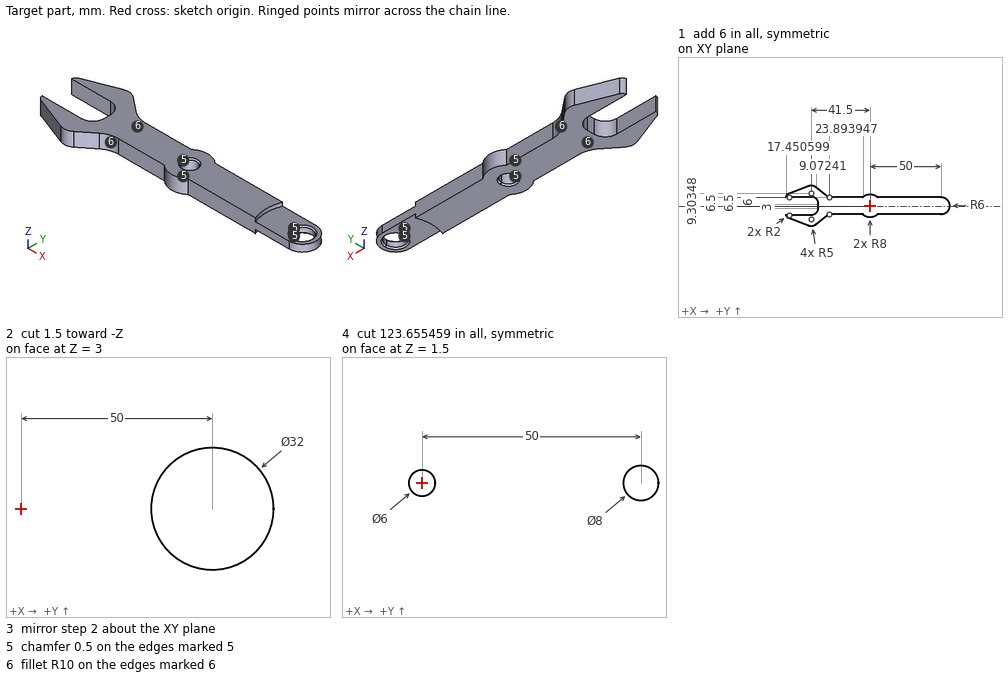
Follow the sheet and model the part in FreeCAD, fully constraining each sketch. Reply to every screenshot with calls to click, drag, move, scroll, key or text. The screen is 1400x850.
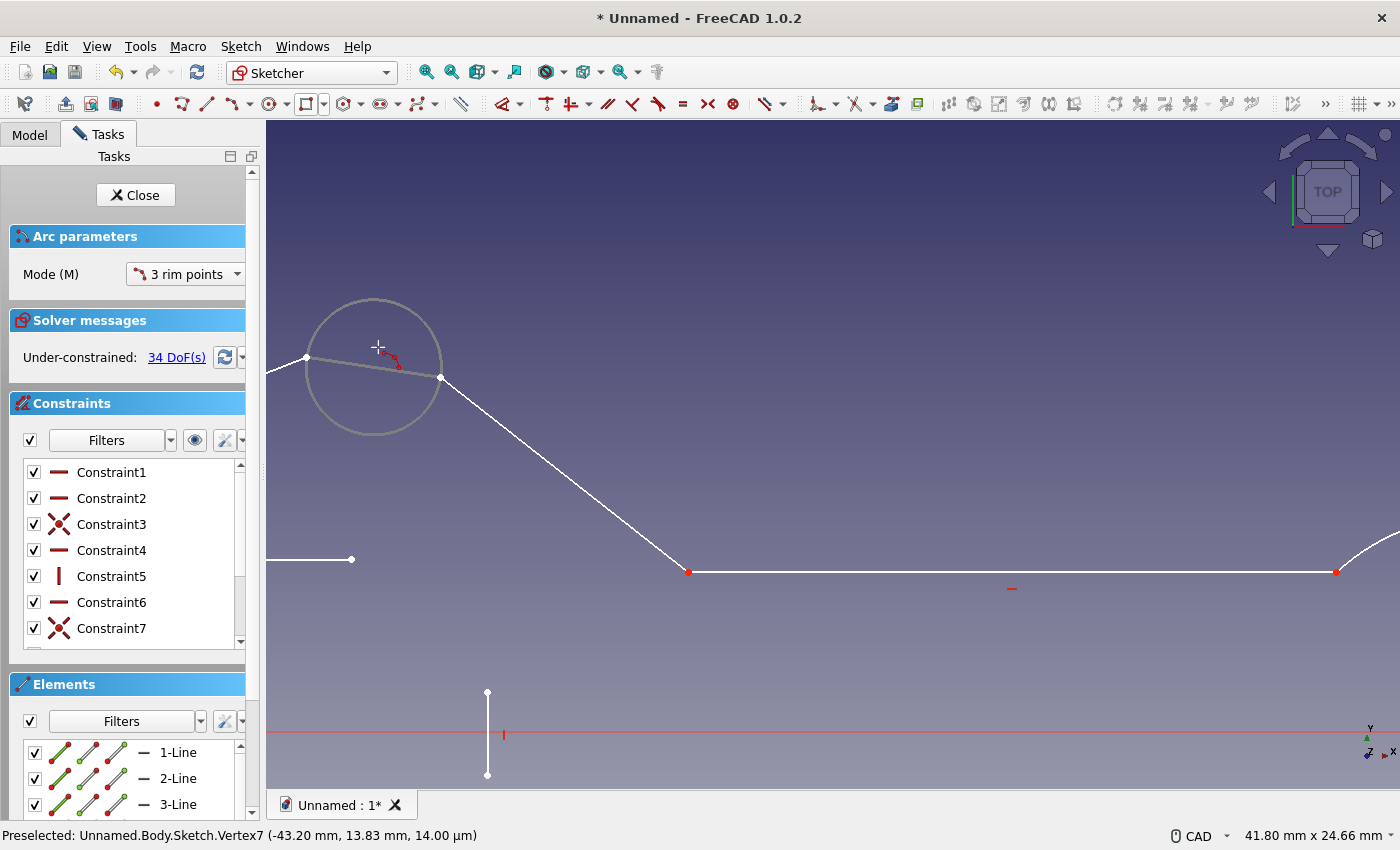
click(377, 346)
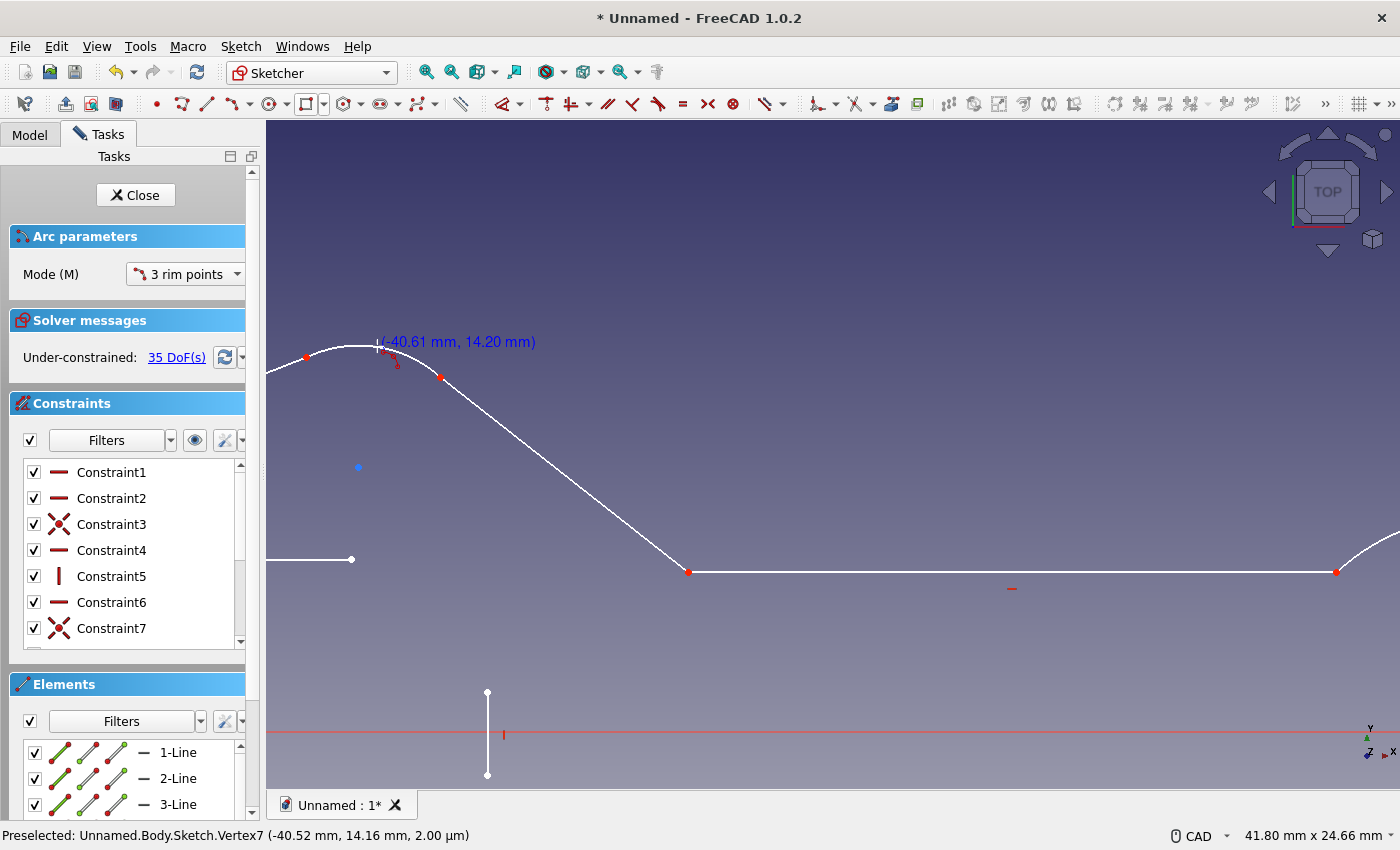
scroll(594, 384, down, 8)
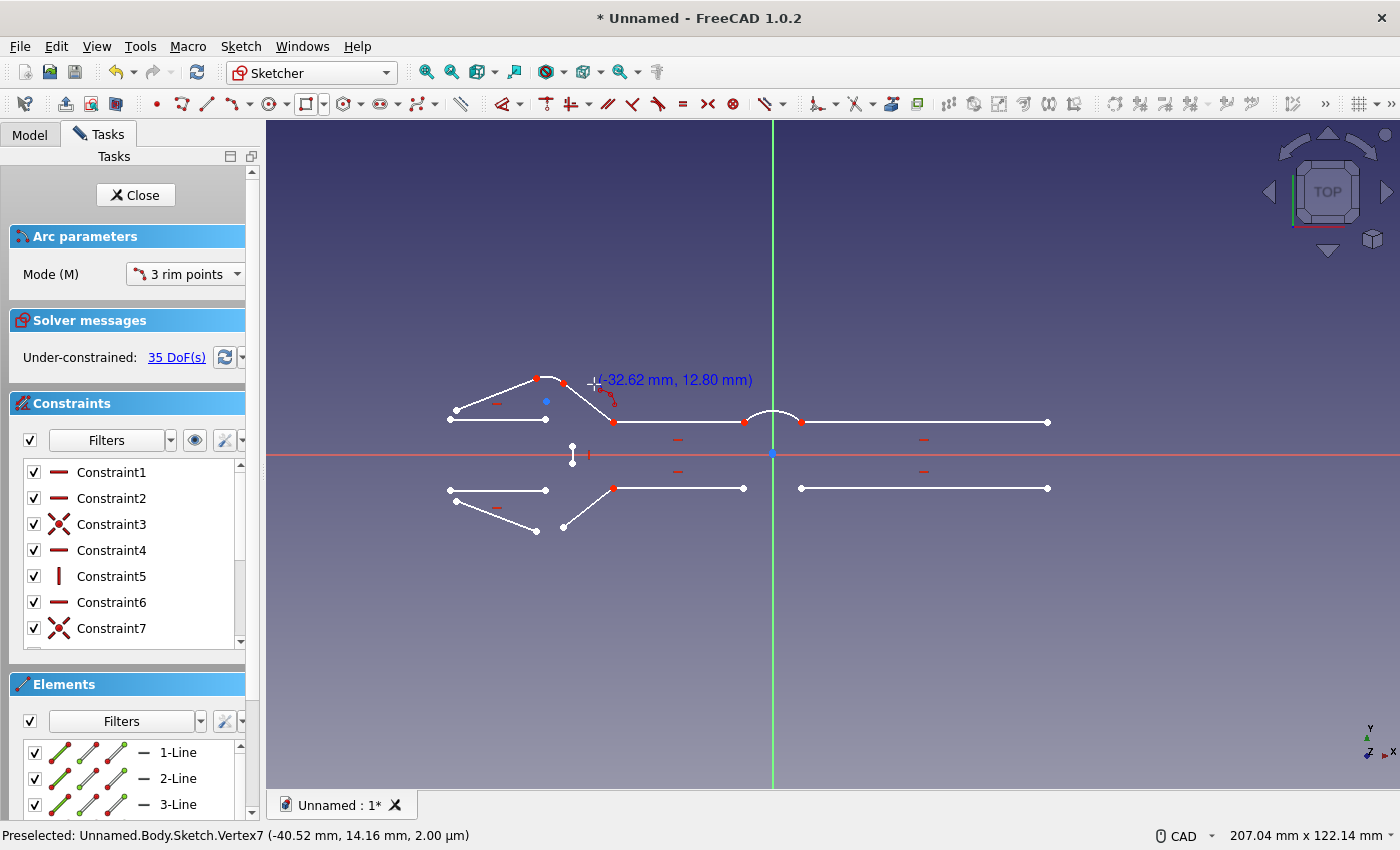
scroll(457, 409, up, 3)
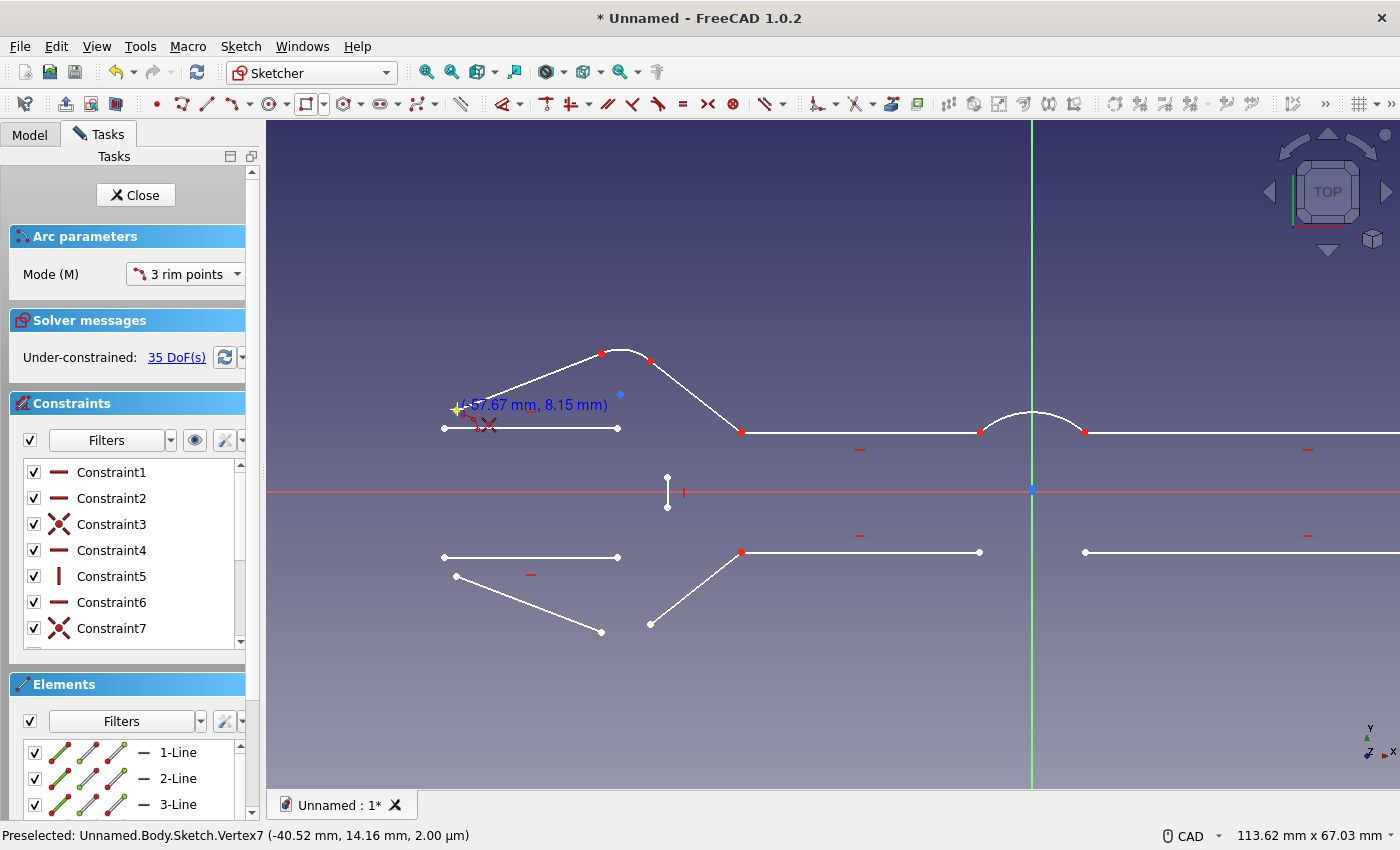
click(457, 411)
click(445, 428)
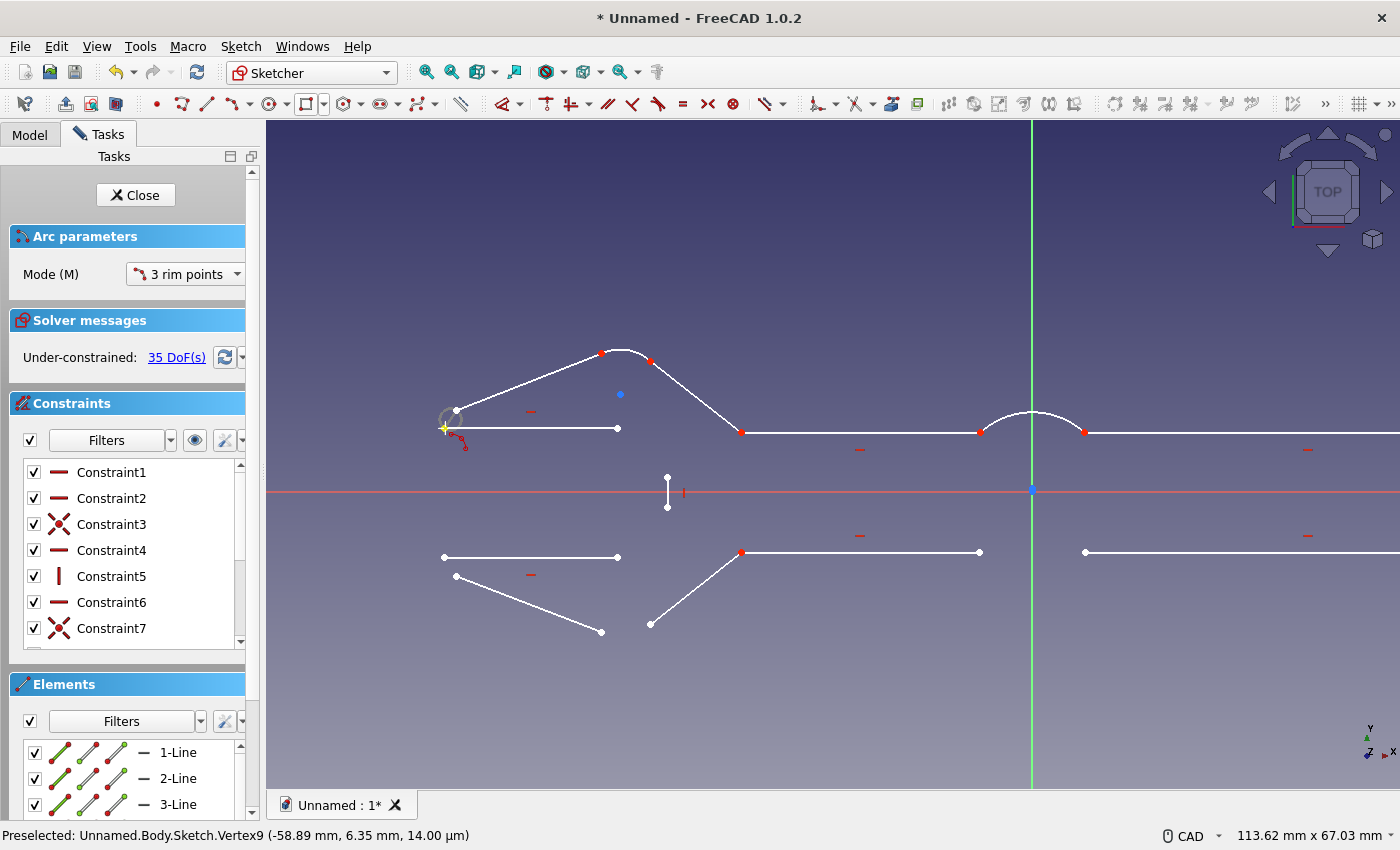
scroll(448, 416, up, 8)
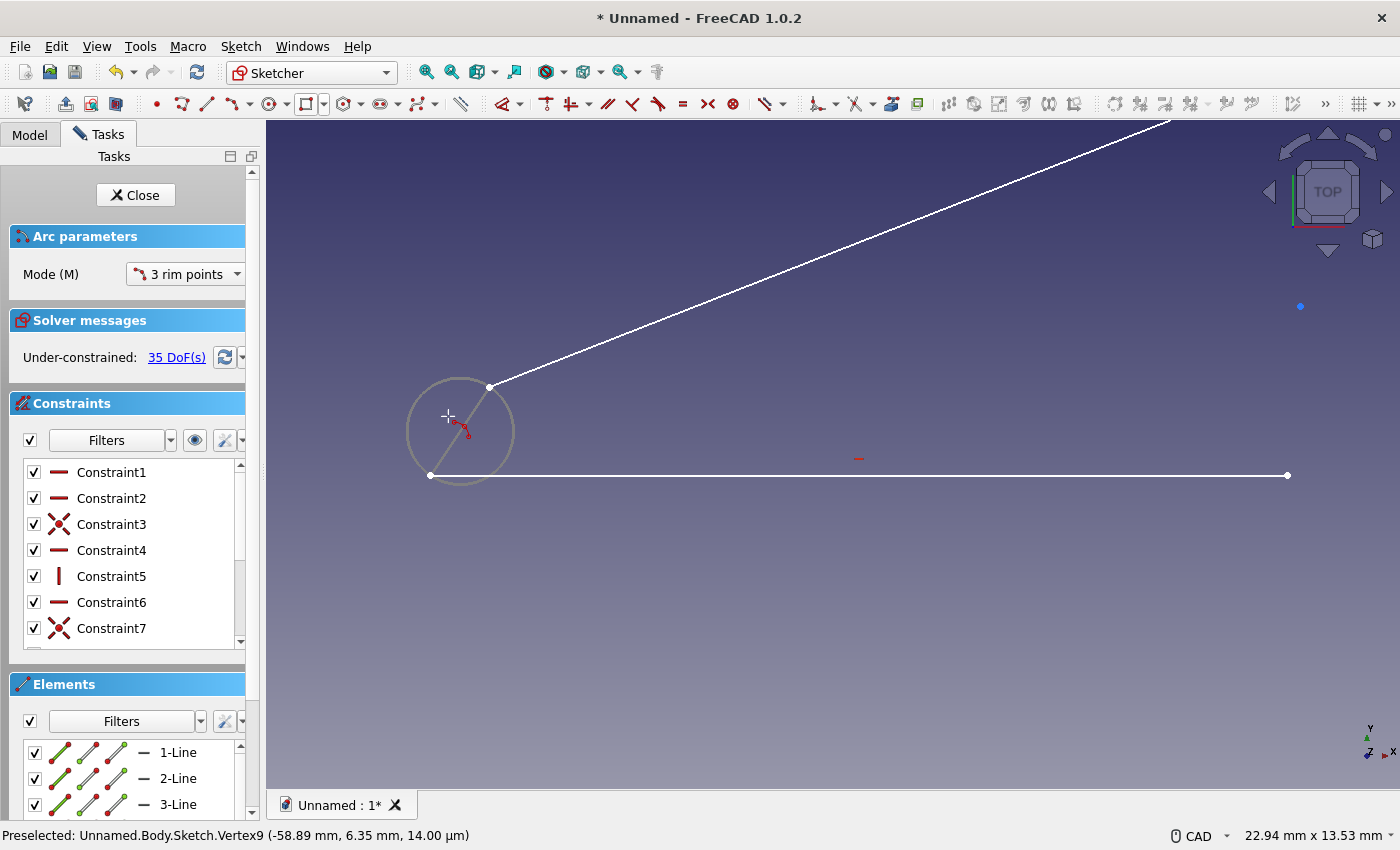
click(445, 413)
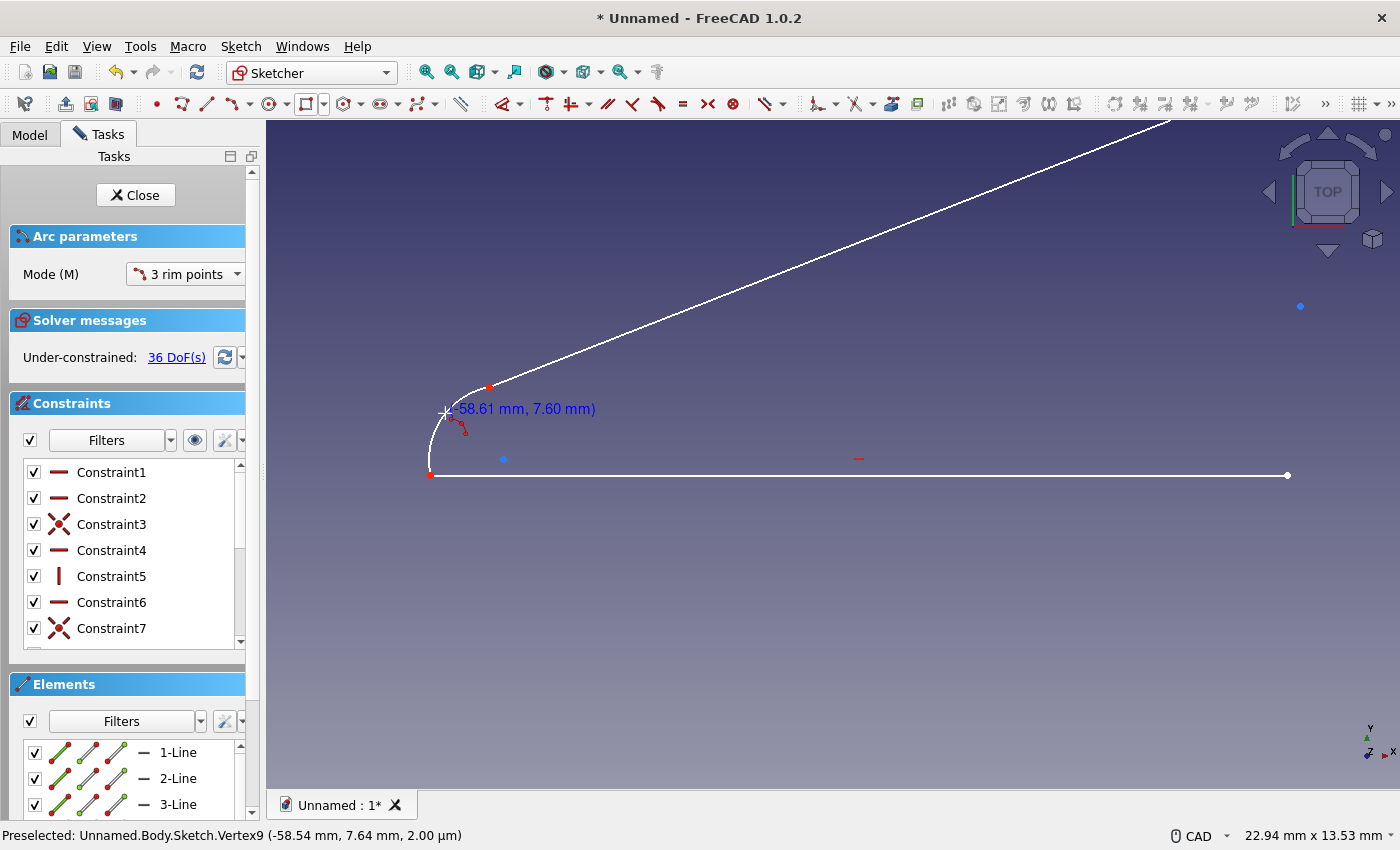
scroll(452, 413, down, 11)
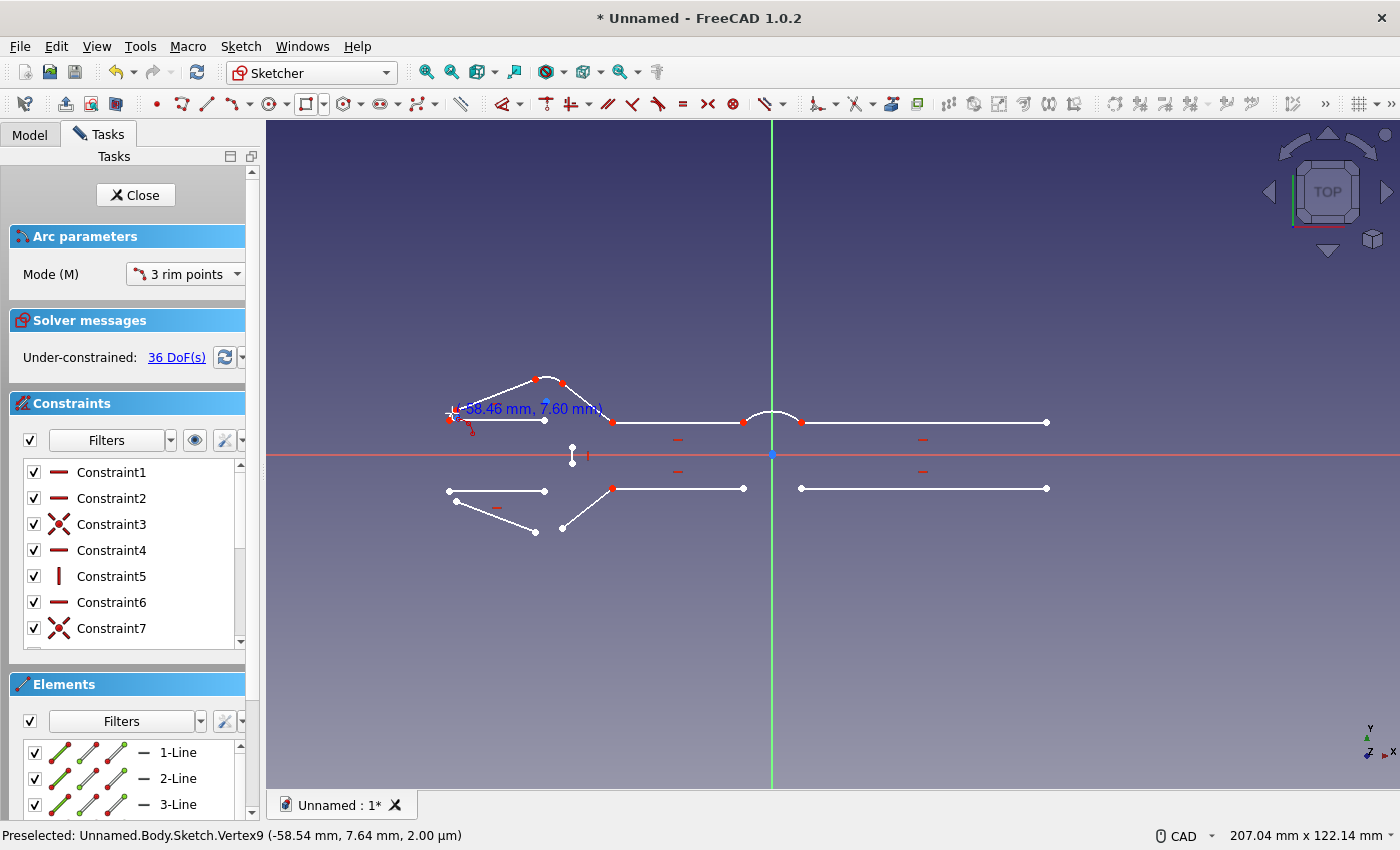
click(545, 420)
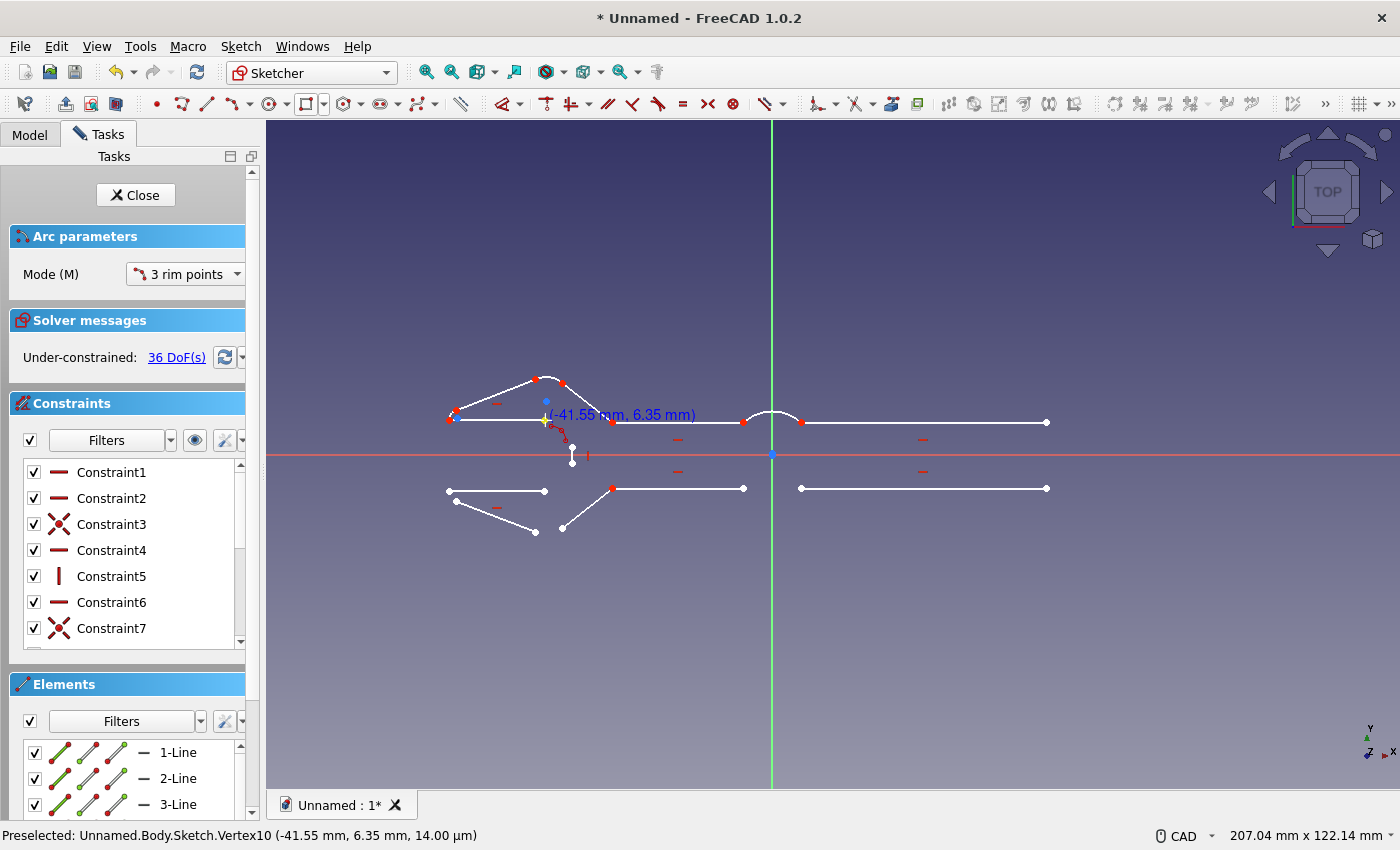
scroll(572, 447, up, 4)